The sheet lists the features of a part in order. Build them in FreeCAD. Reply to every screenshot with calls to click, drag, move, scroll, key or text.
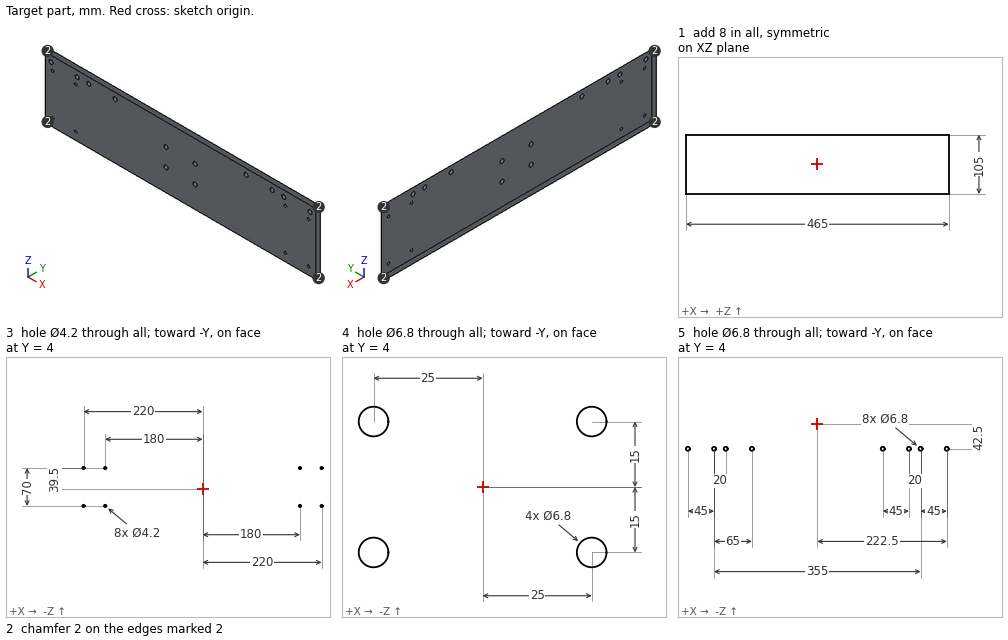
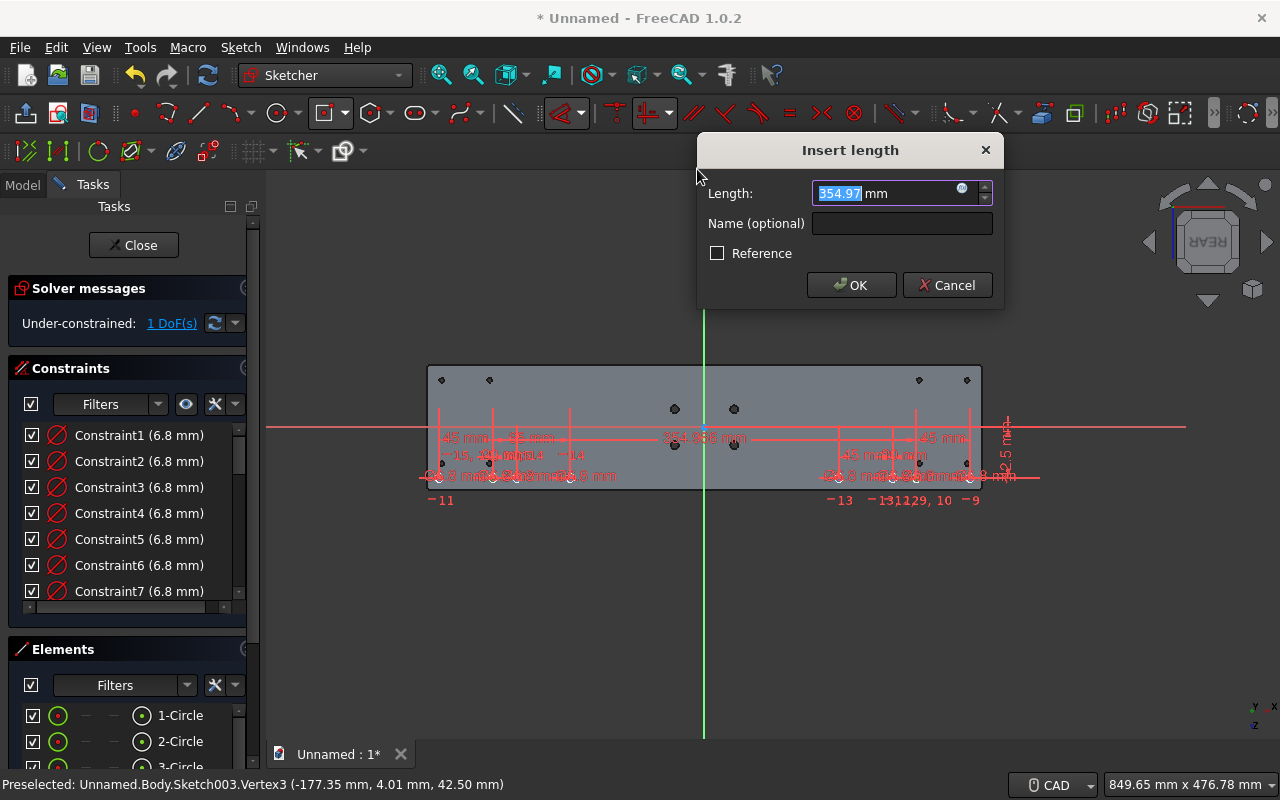
text(355)
key(Return)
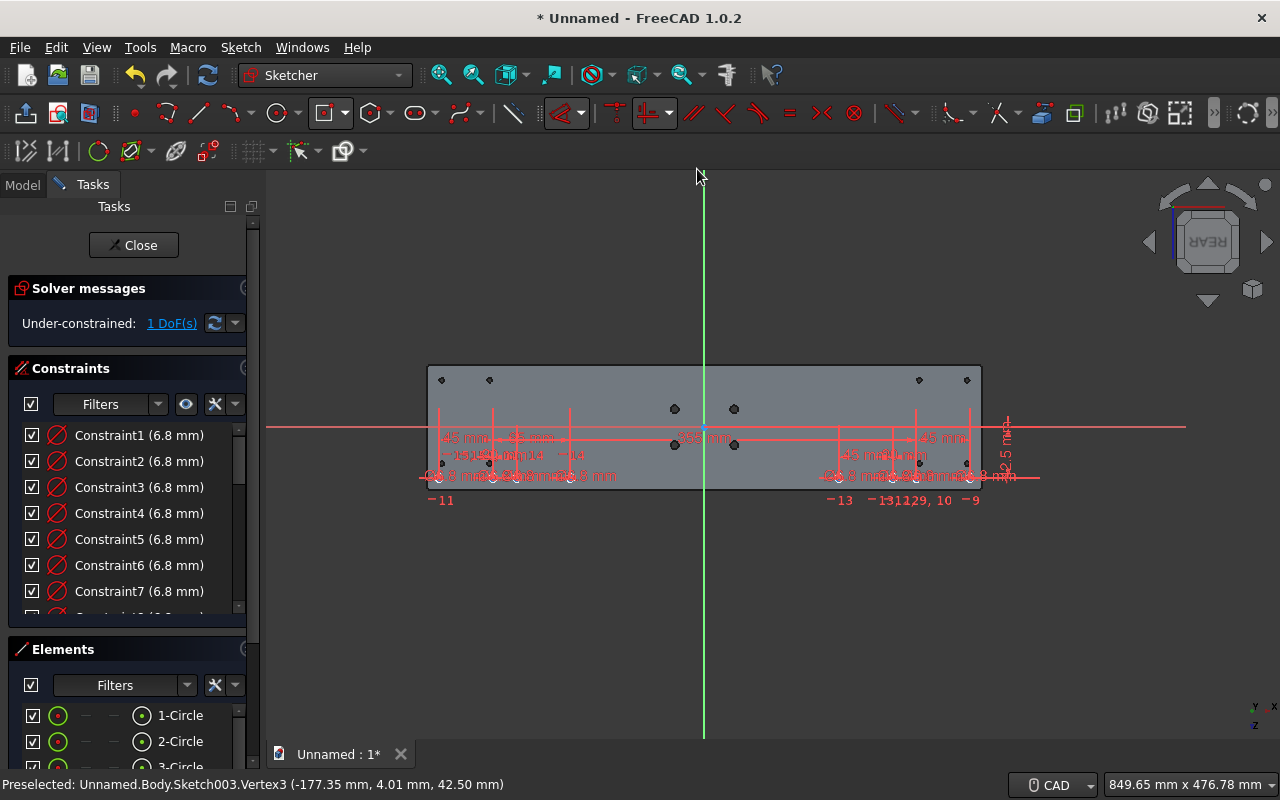
click(970, 478)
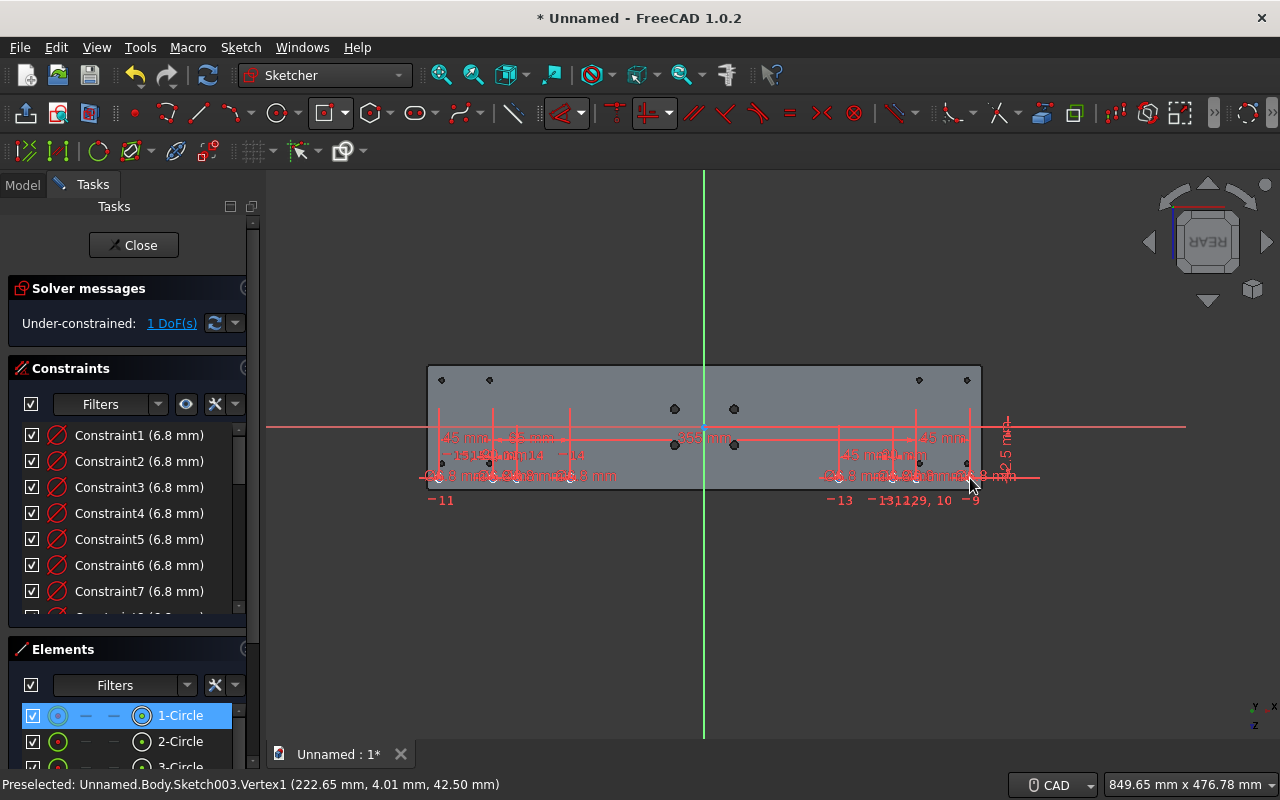
click(584, 114)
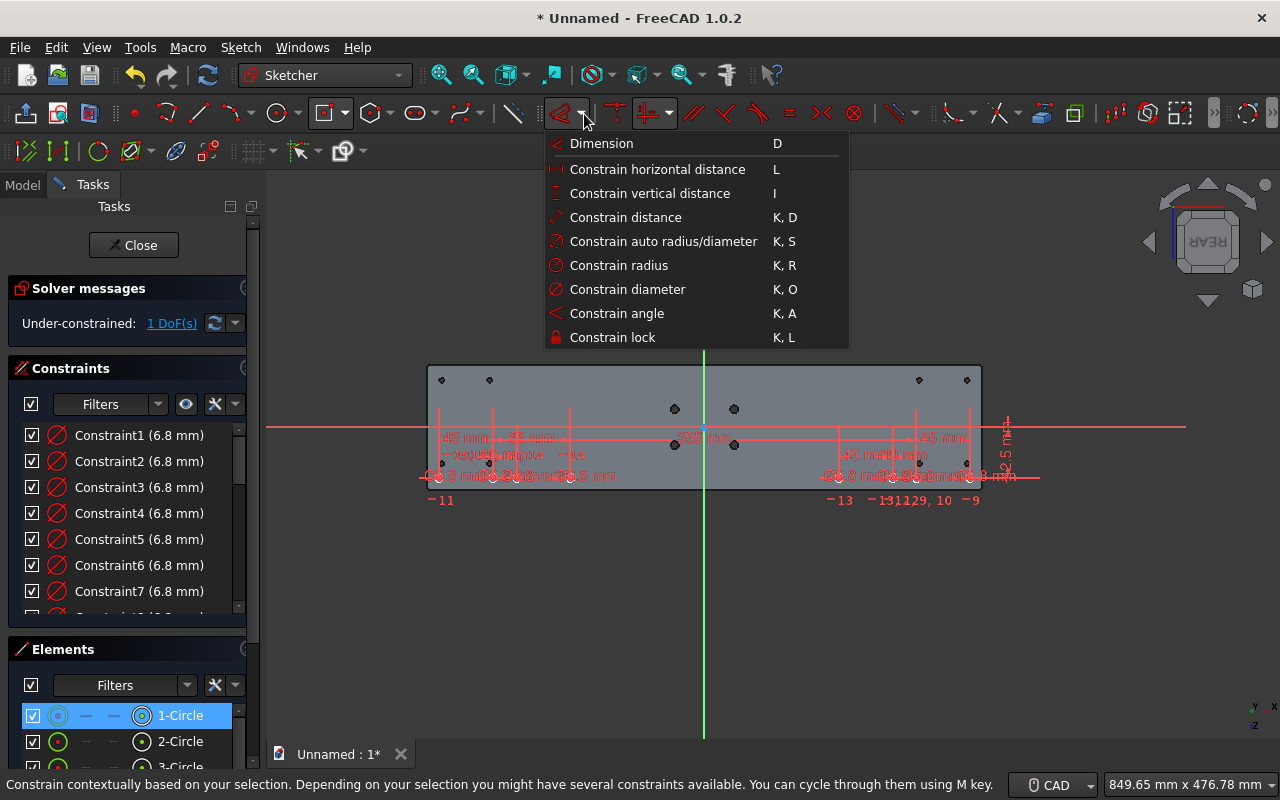
click(697, 169)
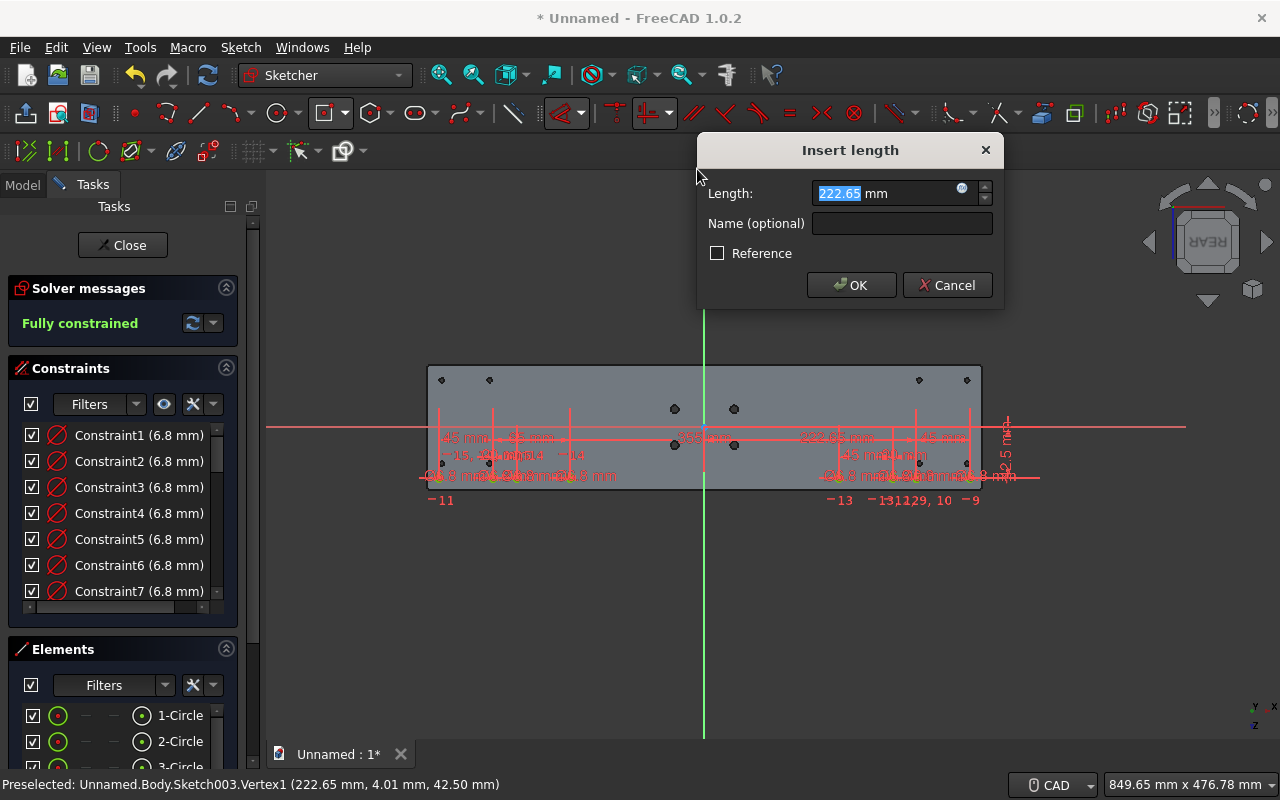
text(222.5)
key(Return)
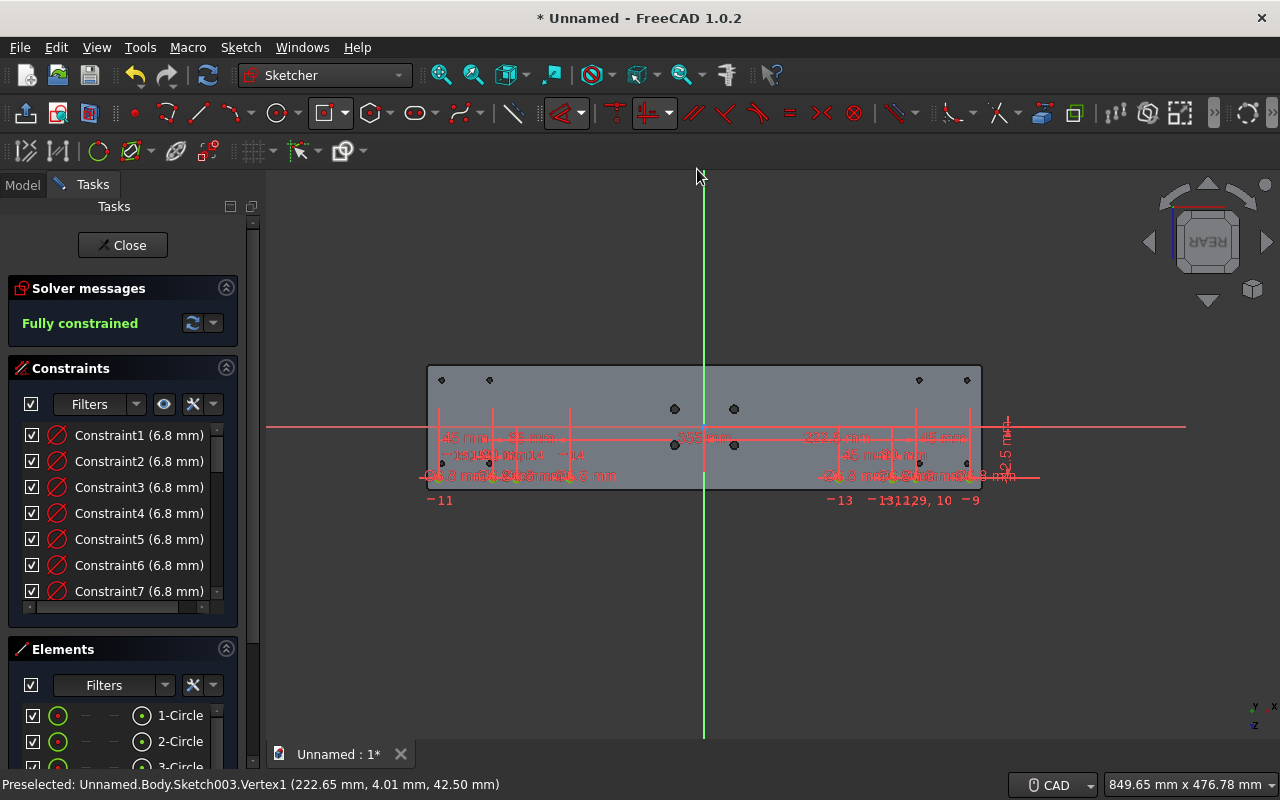
click(123, 245)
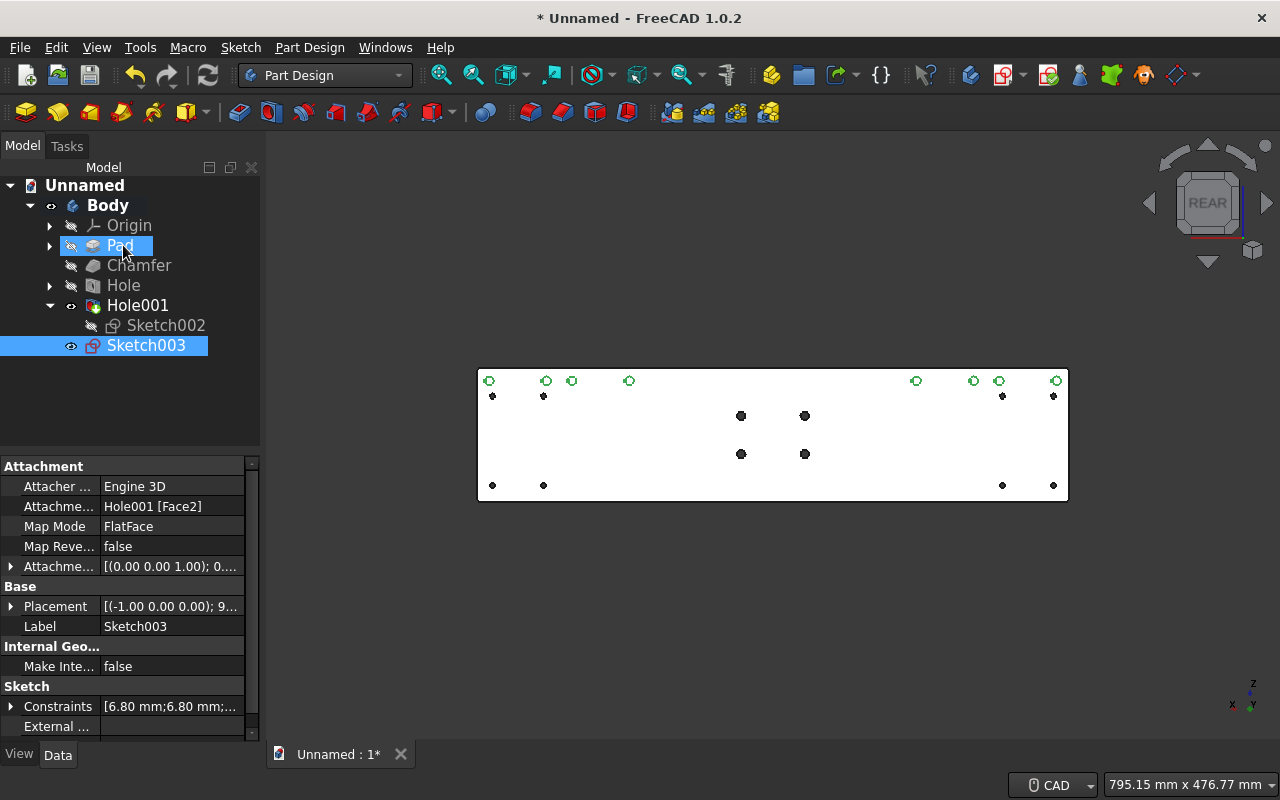
click(272, 112)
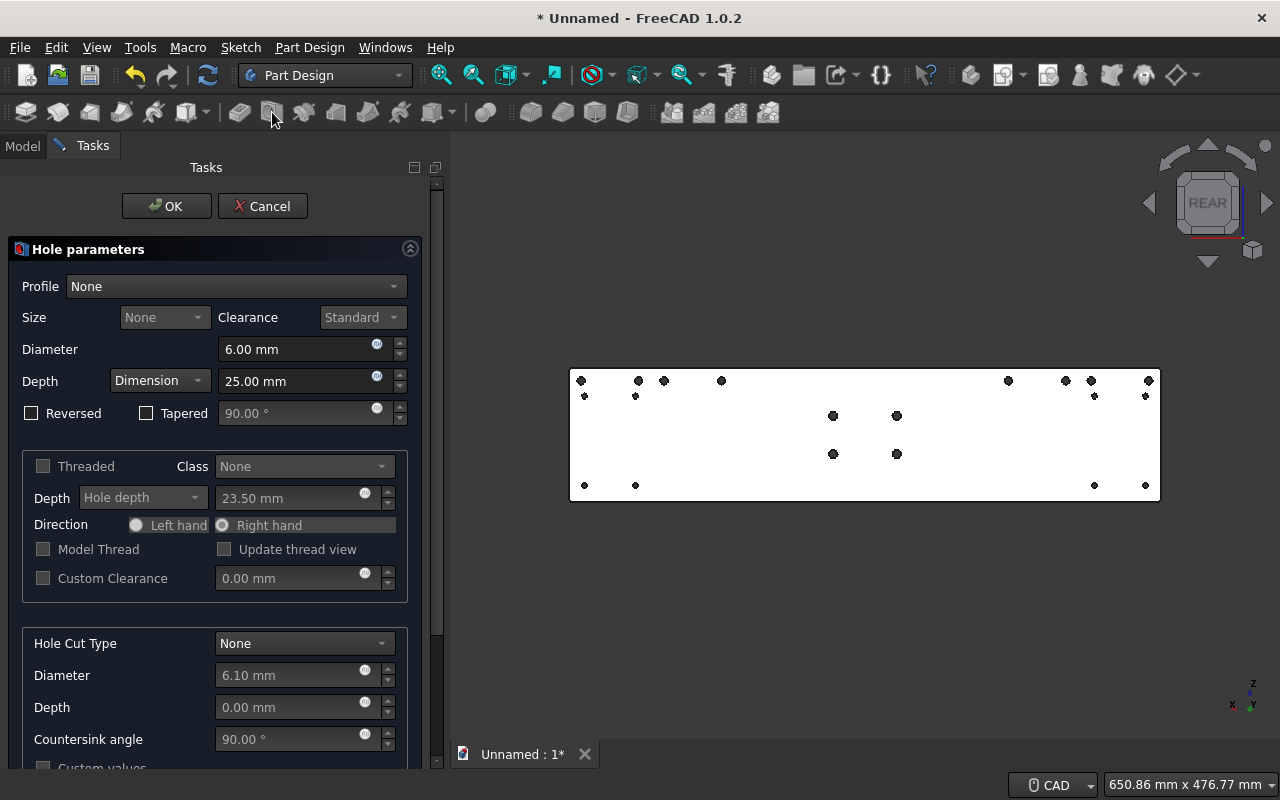
triple_click(305, 349)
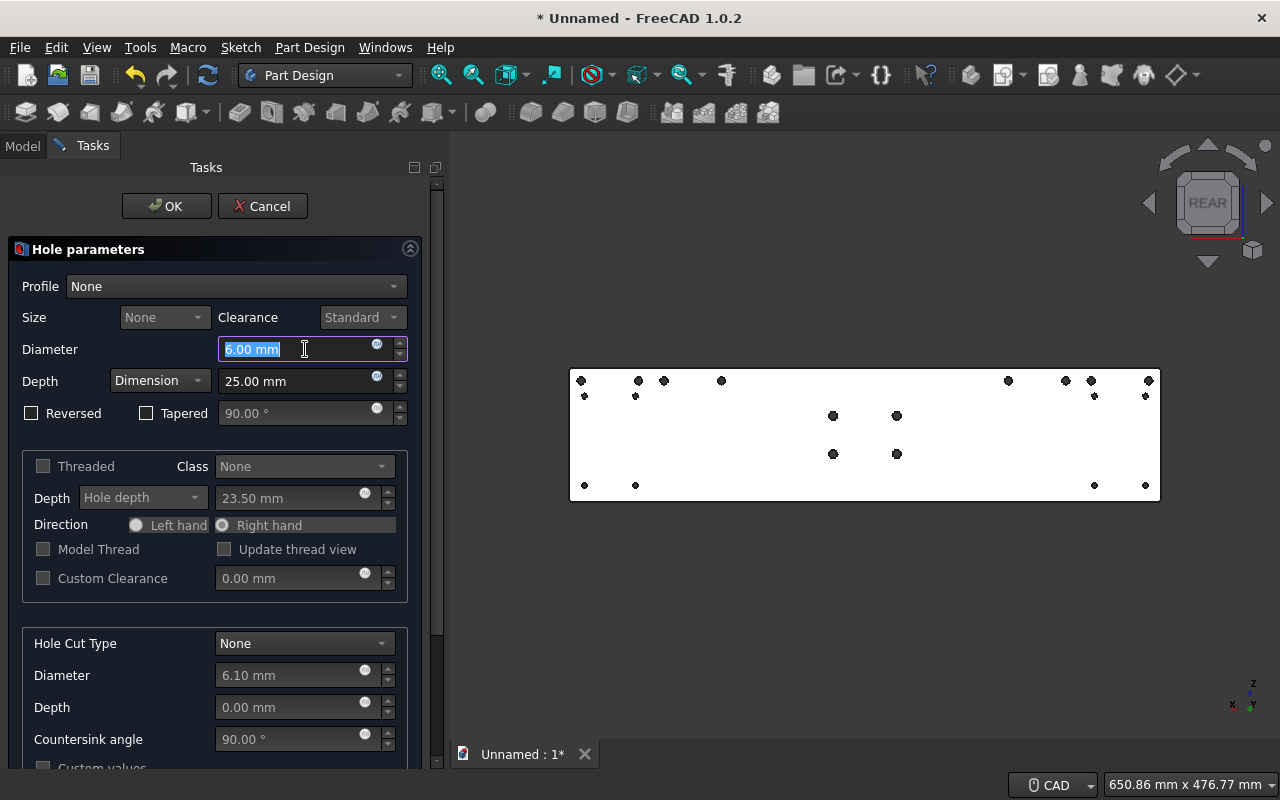
text(6.8)
key(Tab)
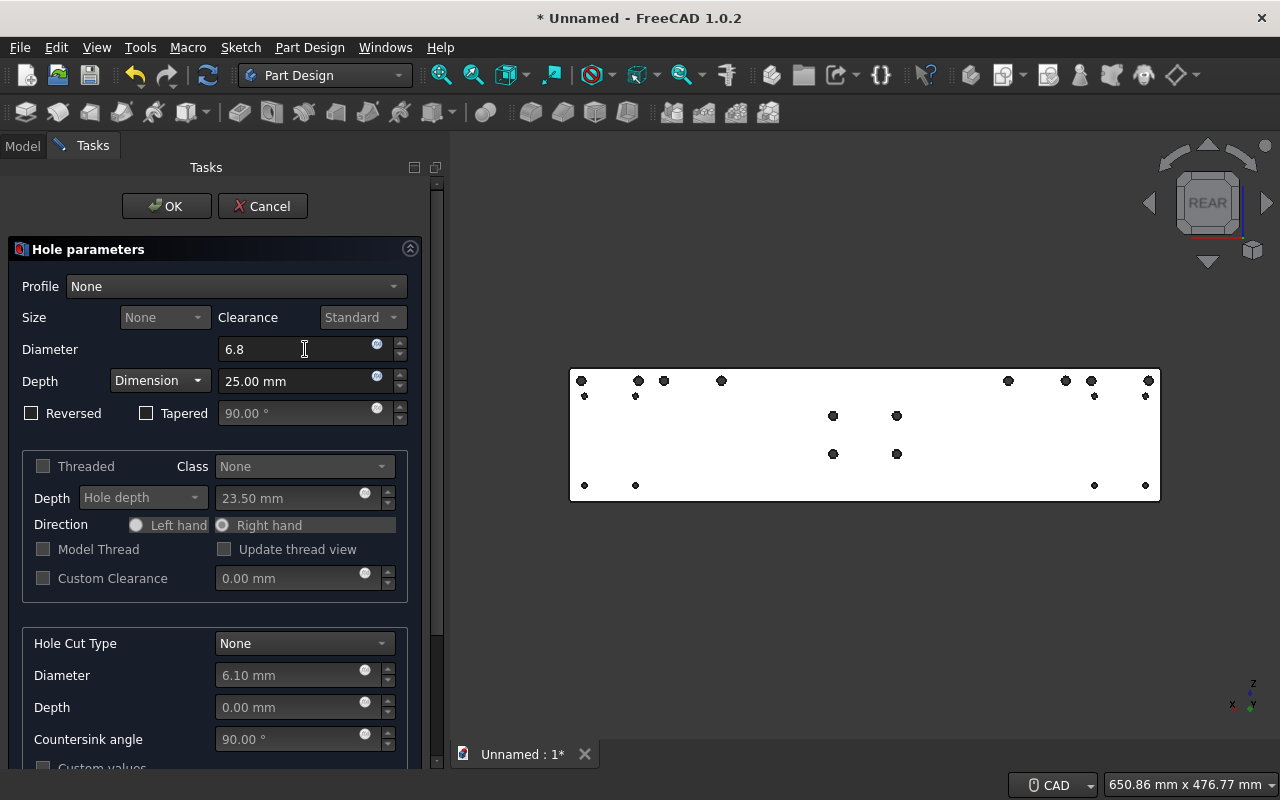
click(161, 380)